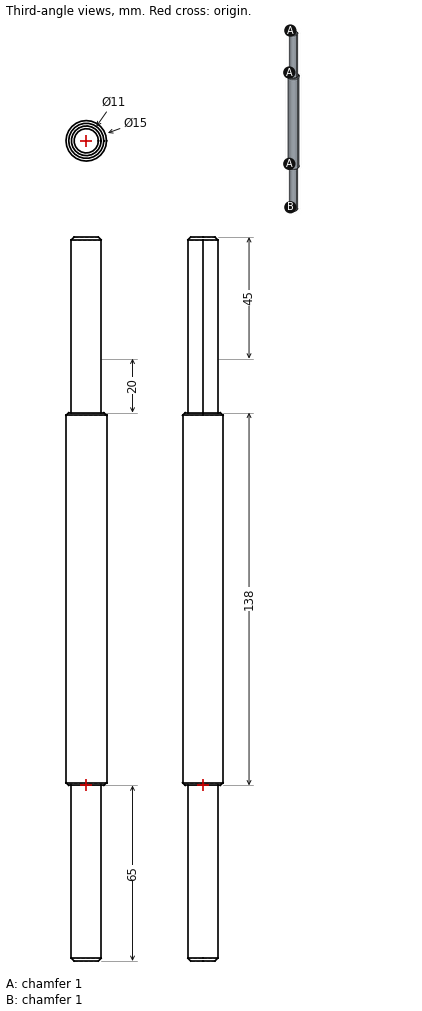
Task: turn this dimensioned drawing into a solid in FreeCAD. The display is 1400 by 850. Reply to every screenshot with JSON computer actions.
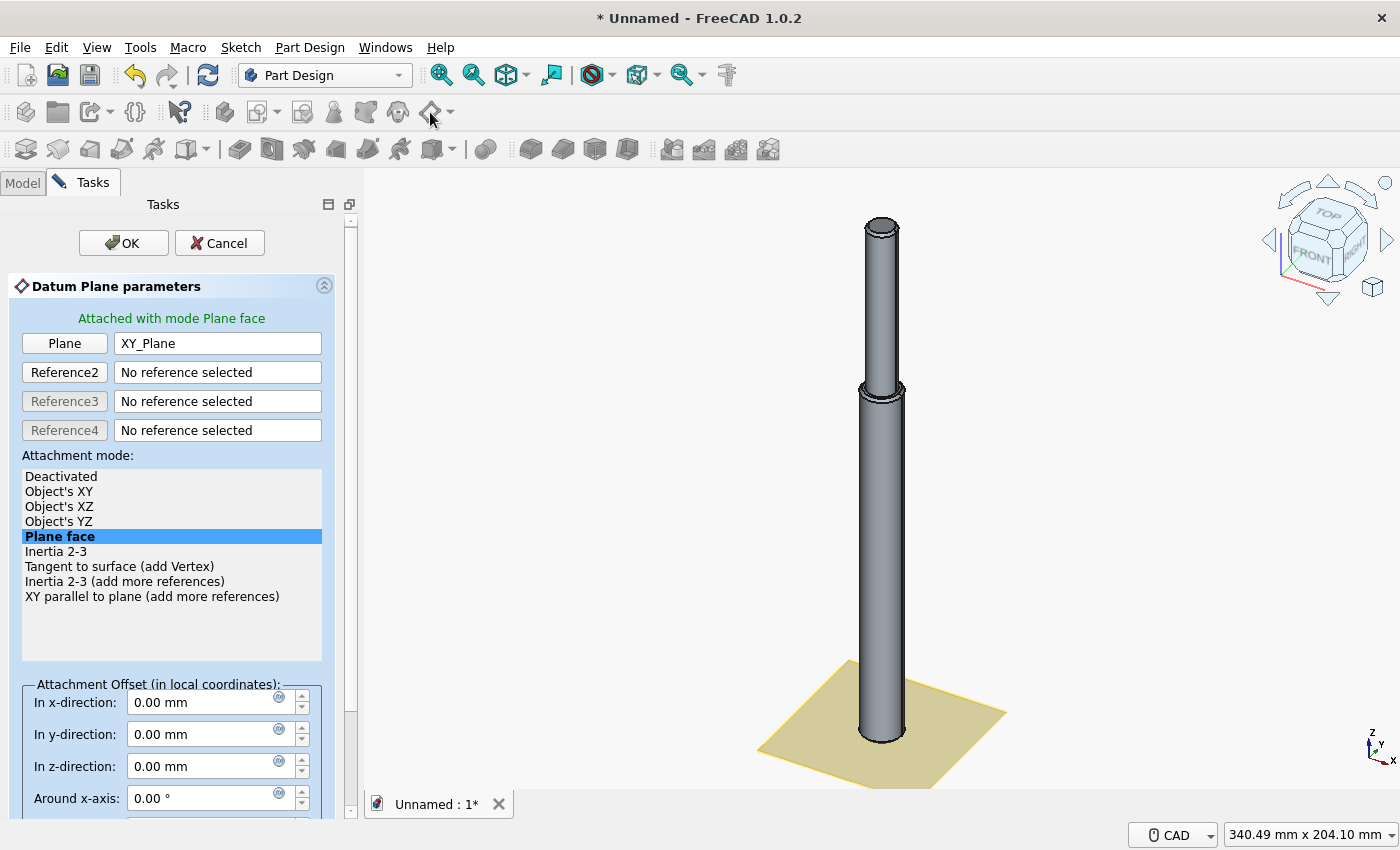
{"action": "triple_click", "coordinate": [210, 766]}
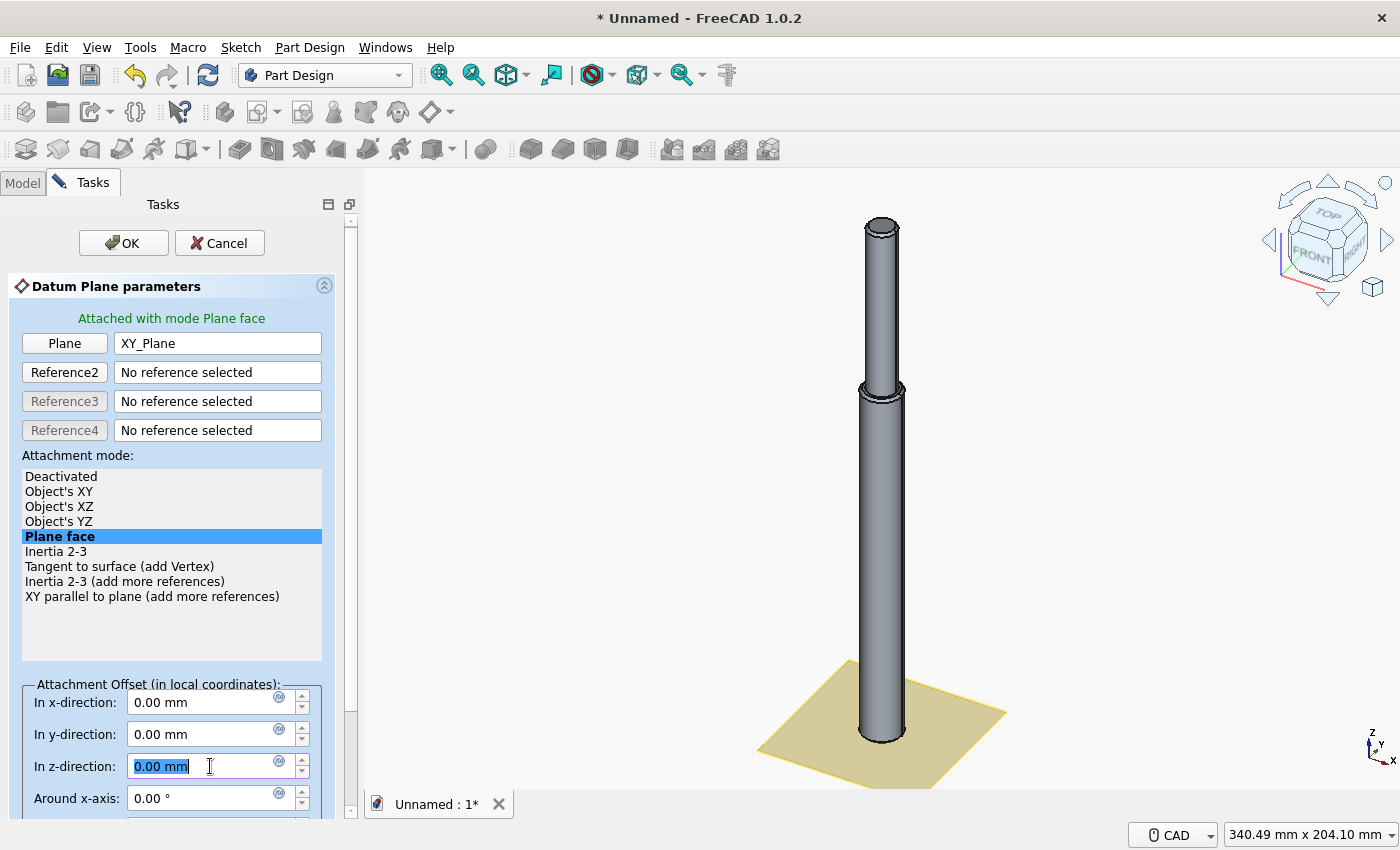
{"action": "type", "text": "-65"}
{"action": "key", "text": "Tab"}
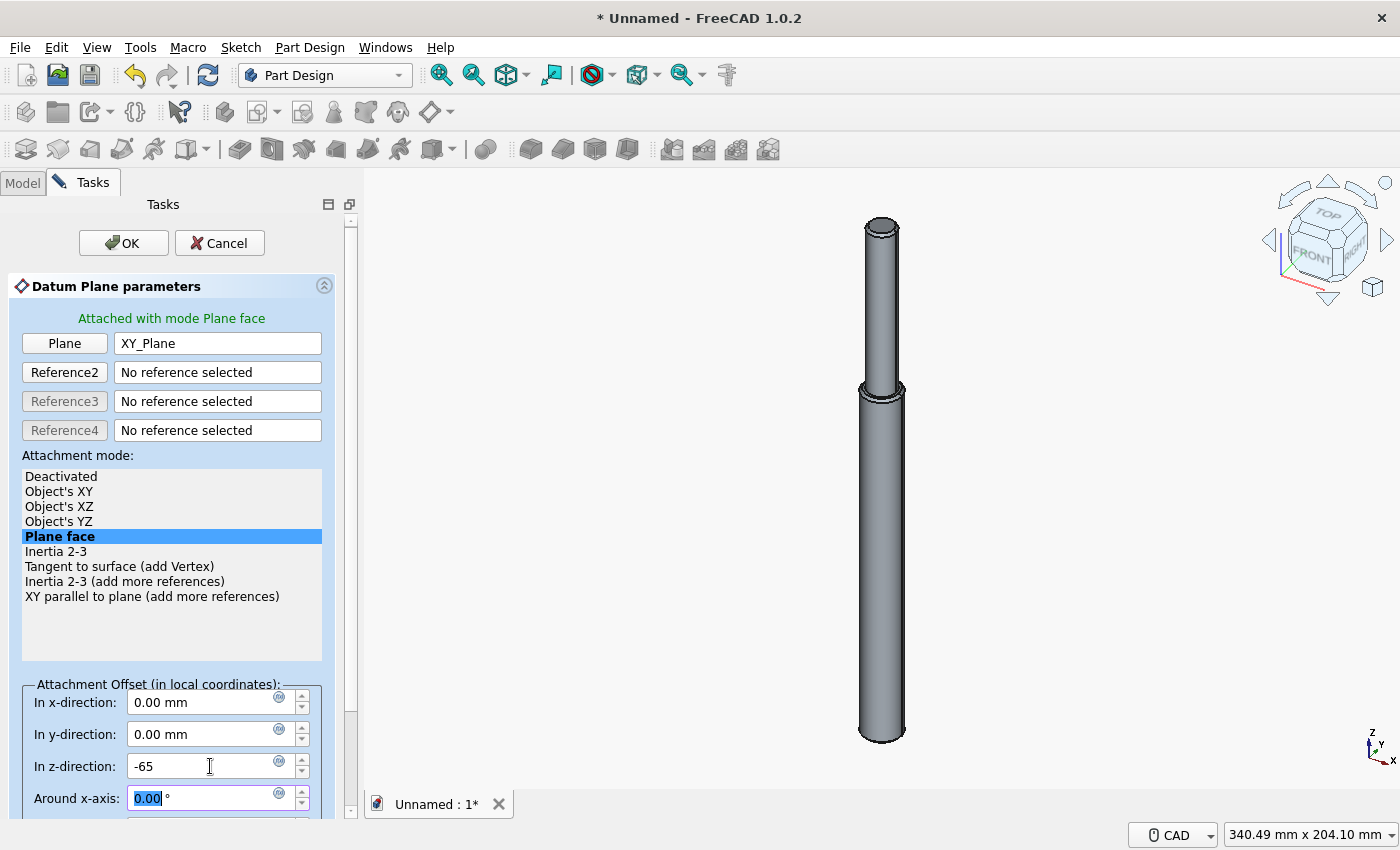
{"action": "left_click", "coordinate": [124, 243]}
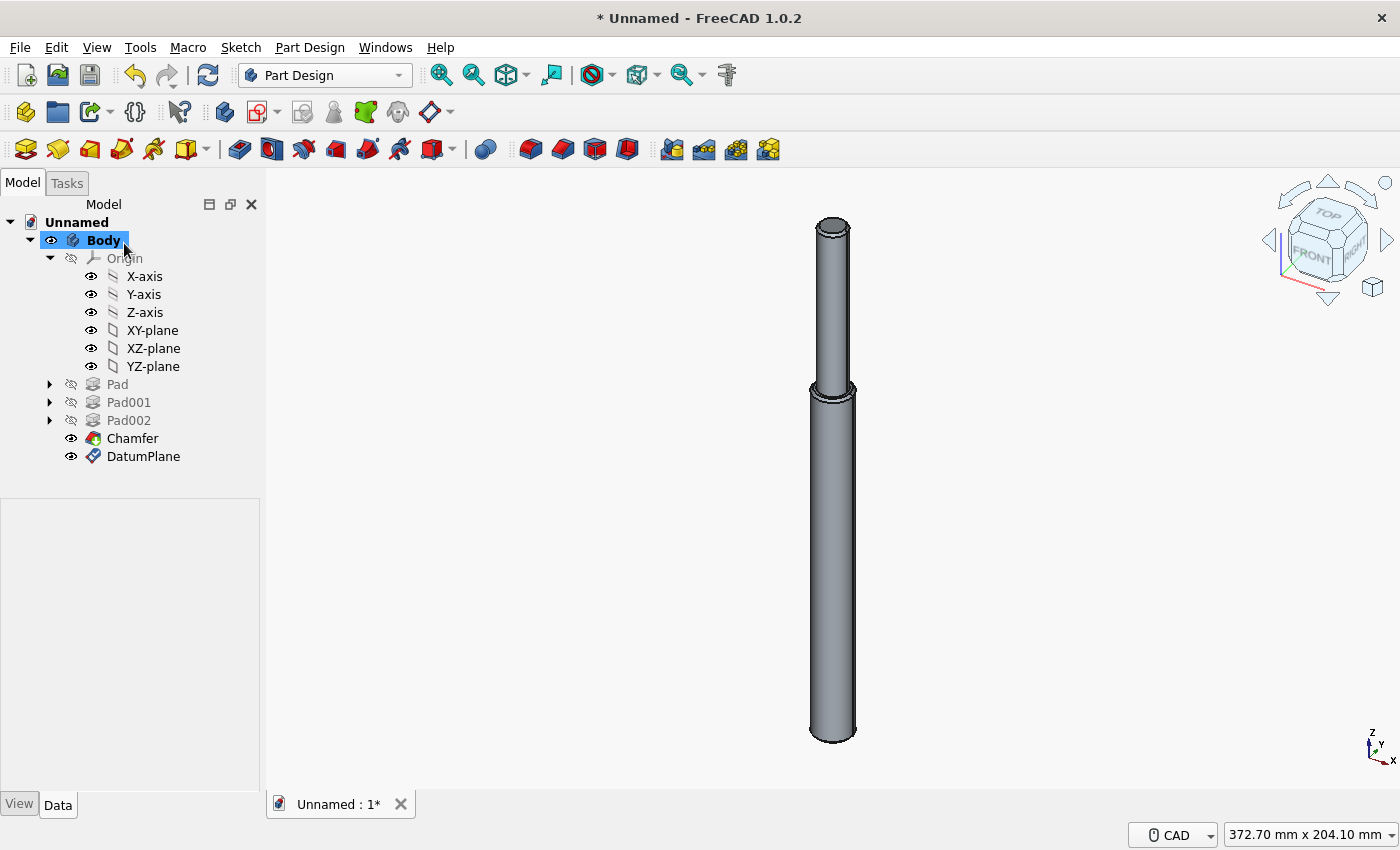
{"action": "left_click", "coordinate": [116, 456]}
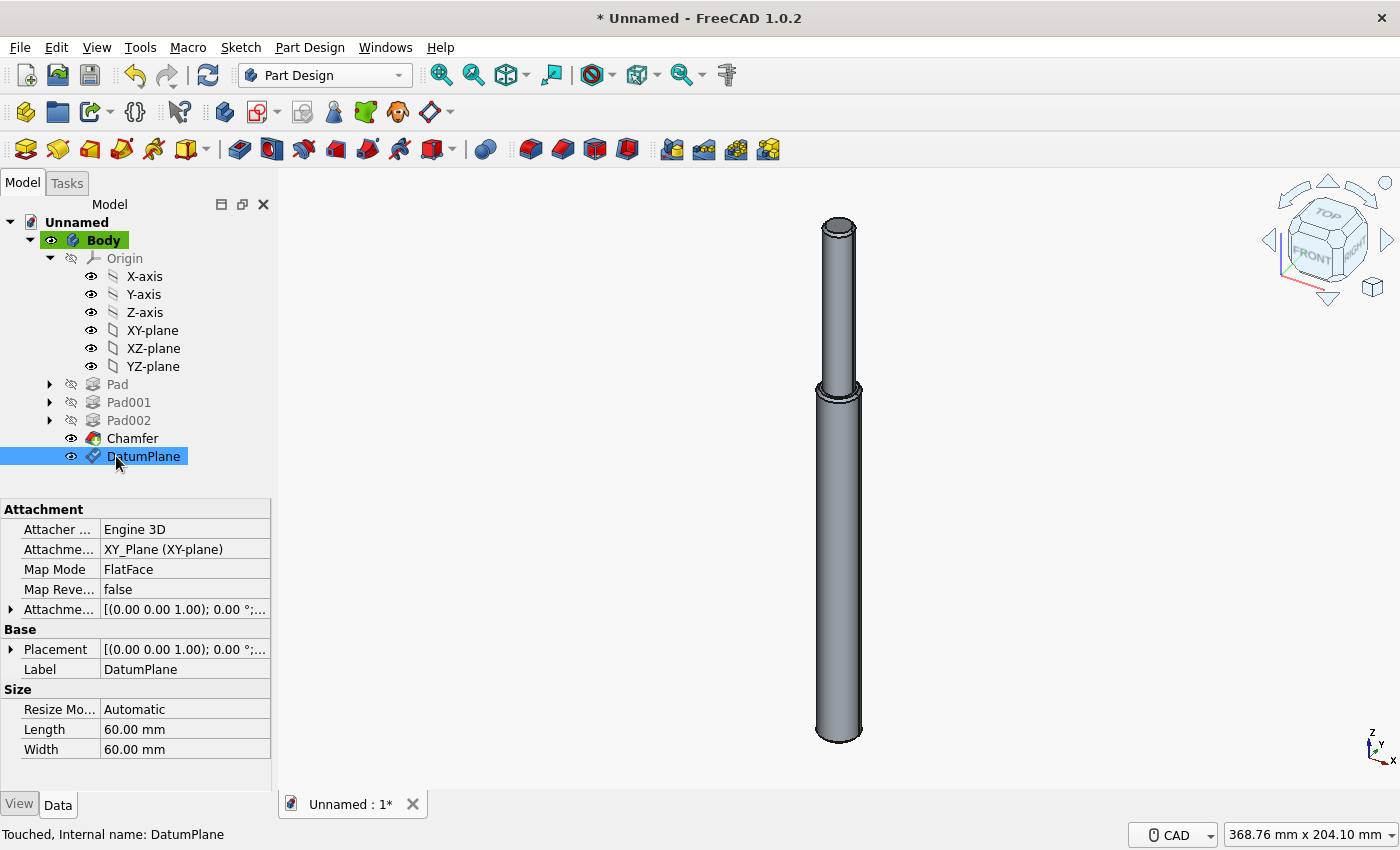
{"action": "left_click", "coordinate": [258, 112]}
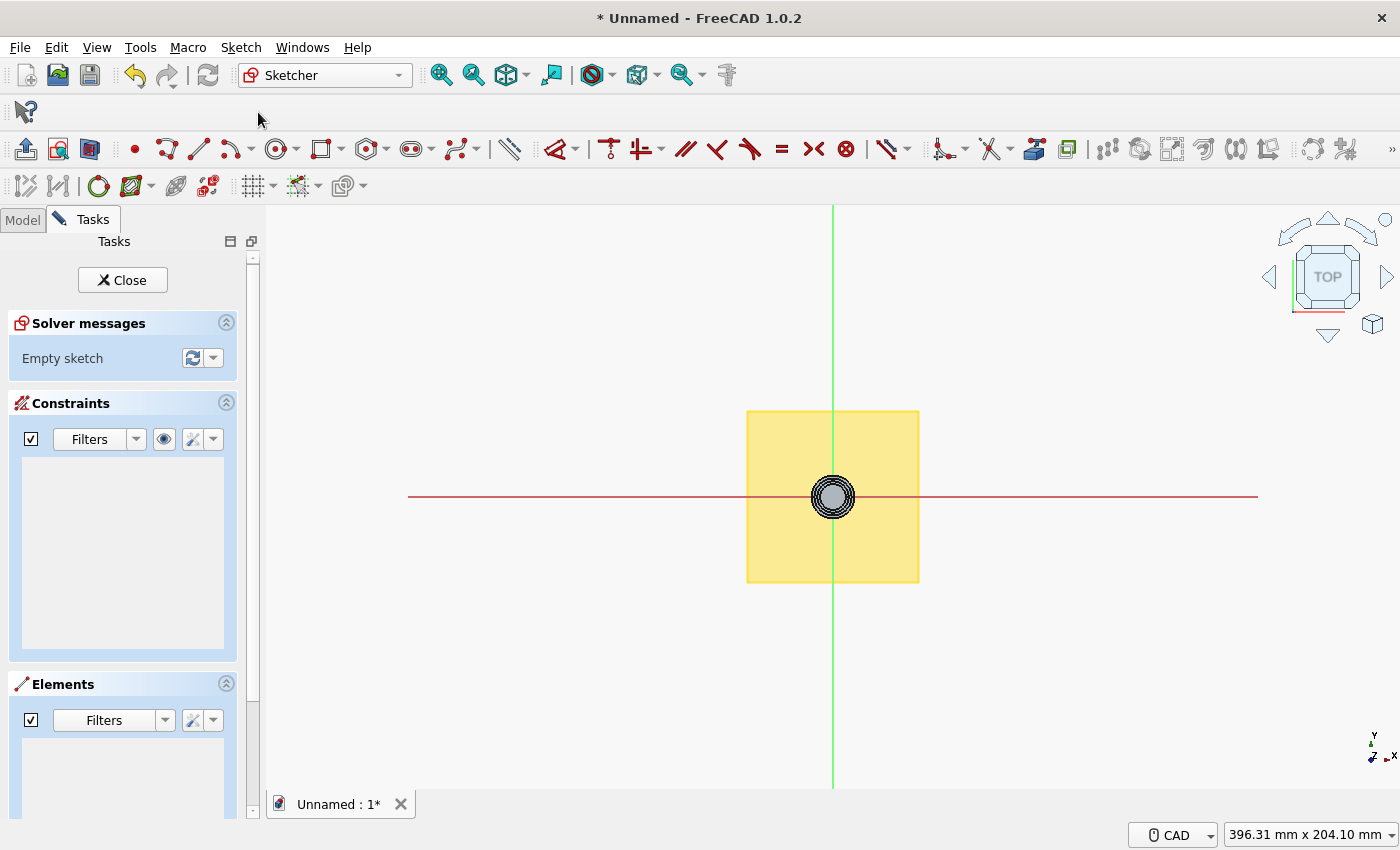
{"action": "key", "text": "q s"}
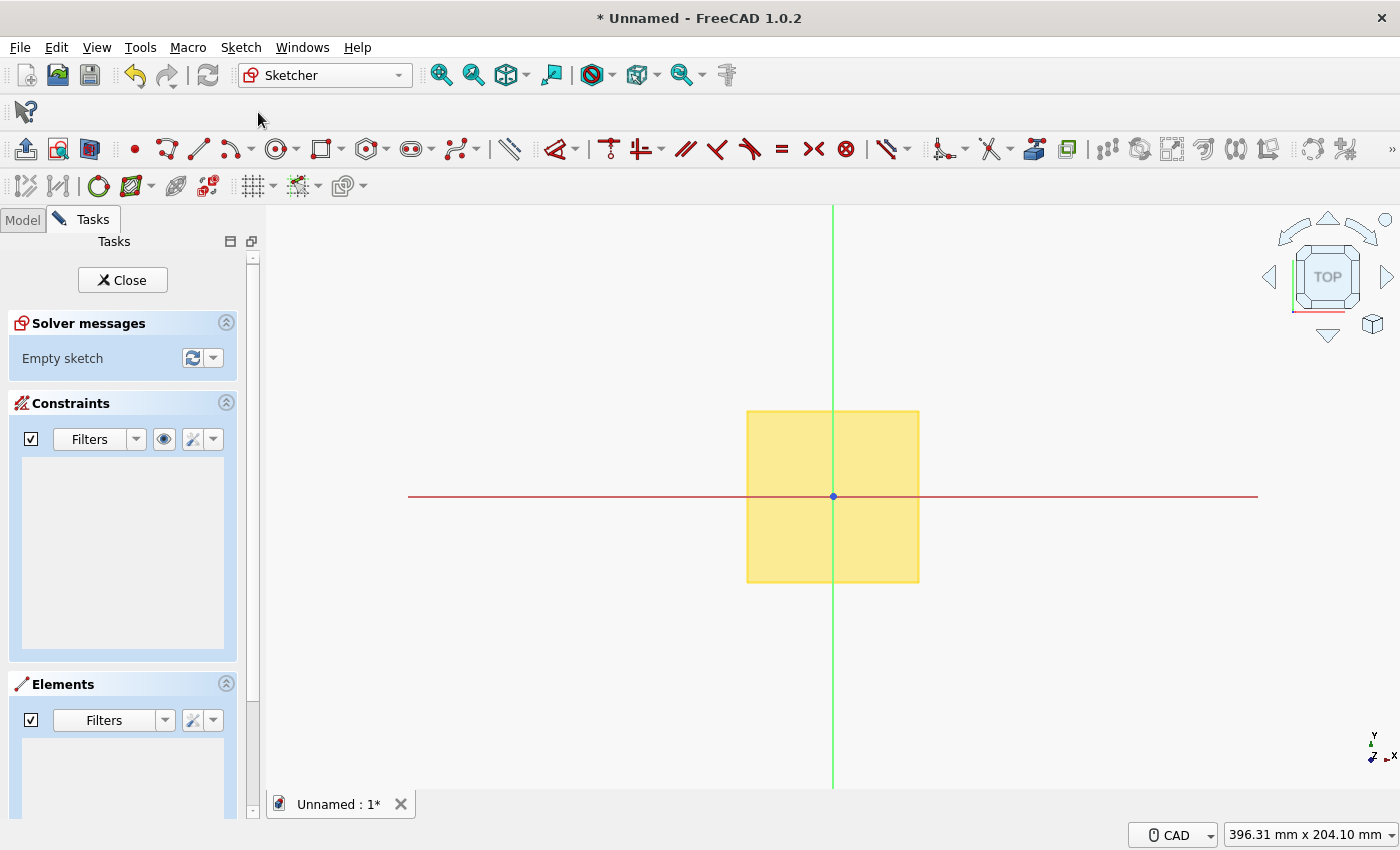
{"action": "scroll", "coordinate": [840, 497], "scroll_direction": "up", "scroll_amount": 12}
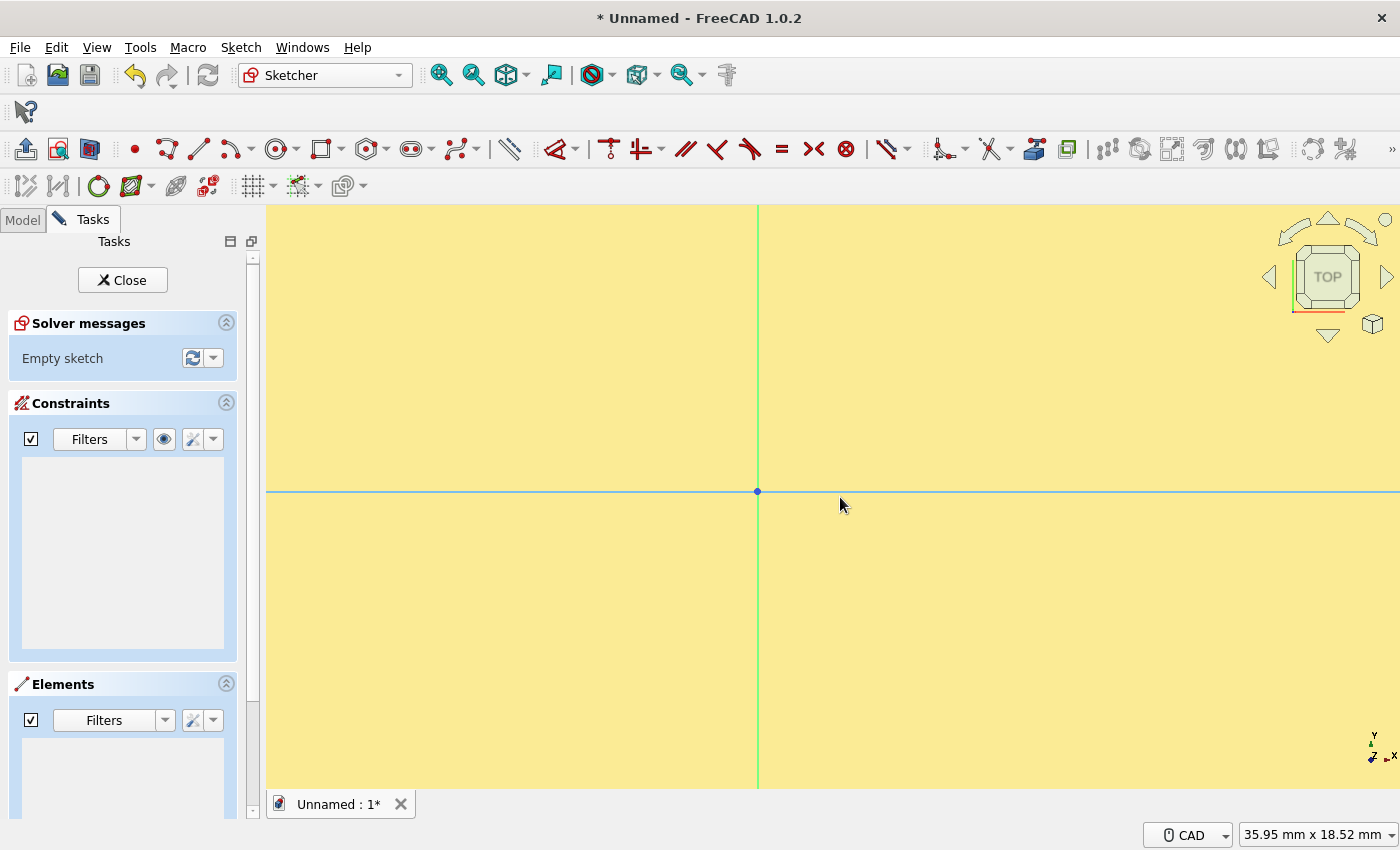
{"action": "key", "text": "g c"}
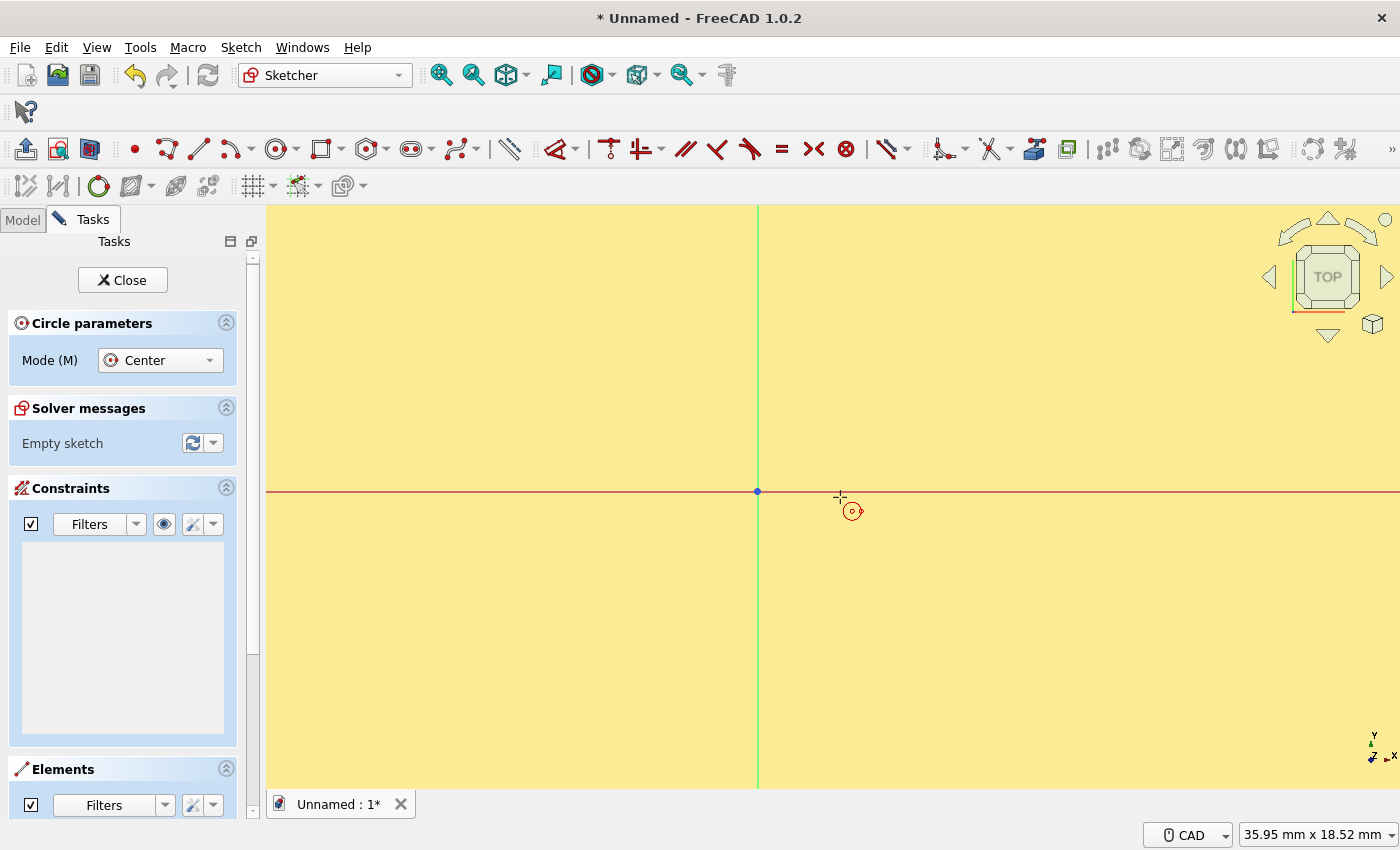
{"action": "left_click", "coordinate": [758, 492]}
{"action": "mouse_move", "coordinate": [880, 369]}